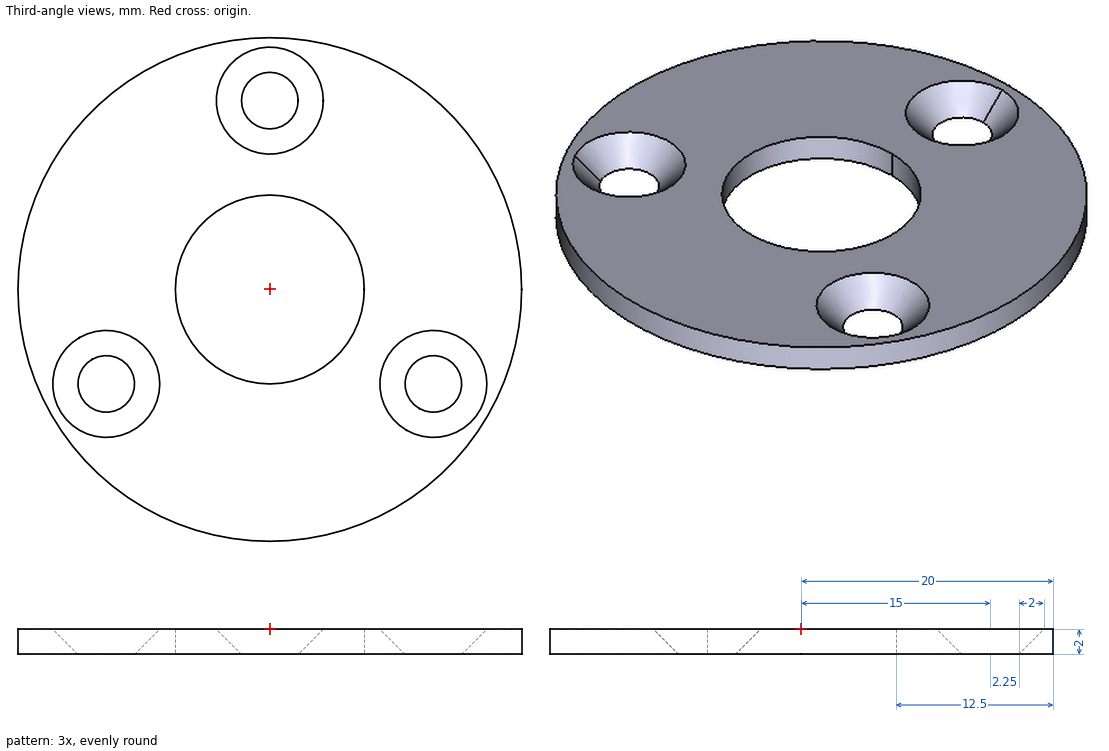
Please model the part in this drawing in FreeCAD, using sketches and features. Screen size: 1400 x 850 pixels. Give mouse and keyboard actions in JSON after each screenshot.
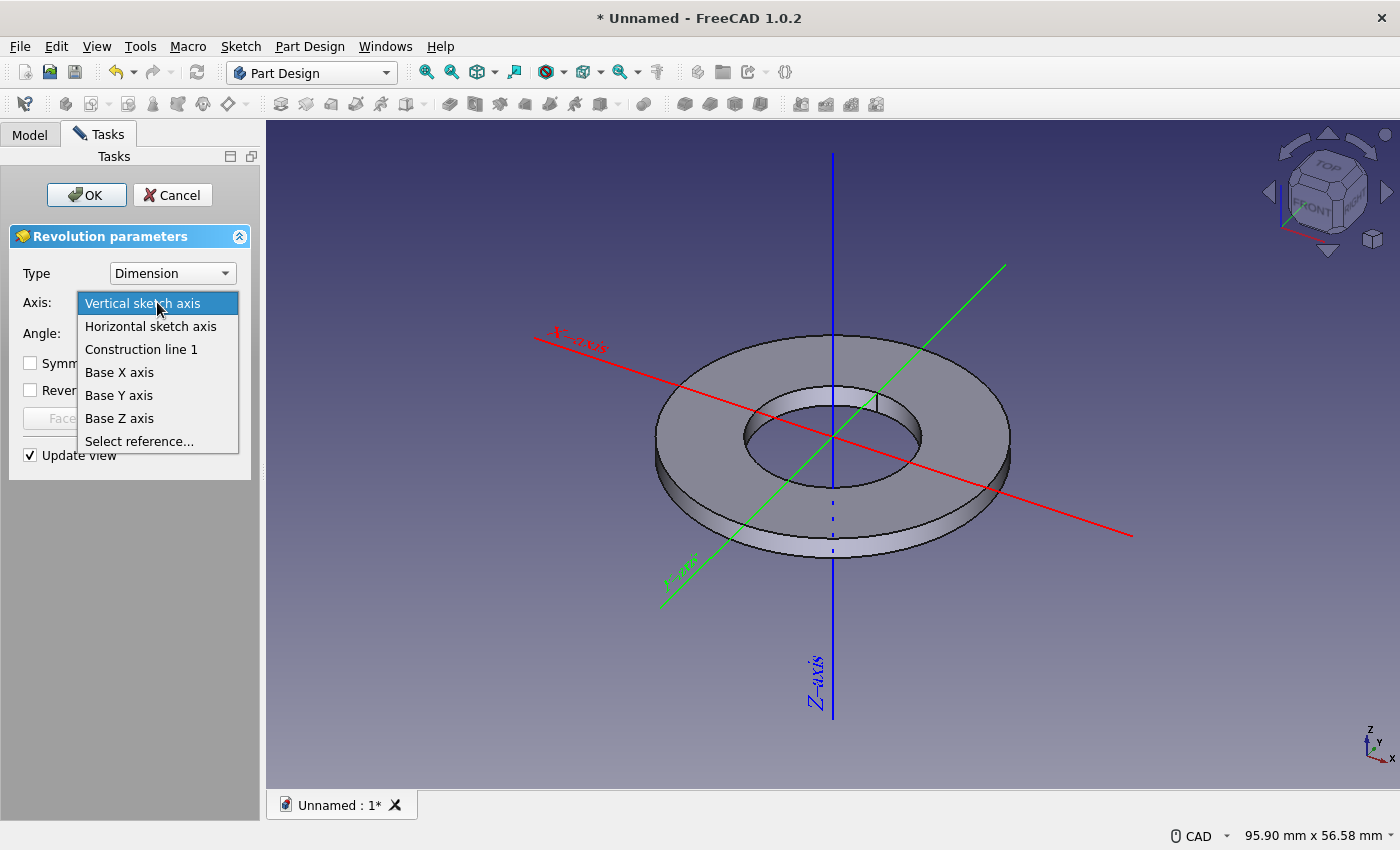
{"action": "left_click", "coordinate": [156, 350]}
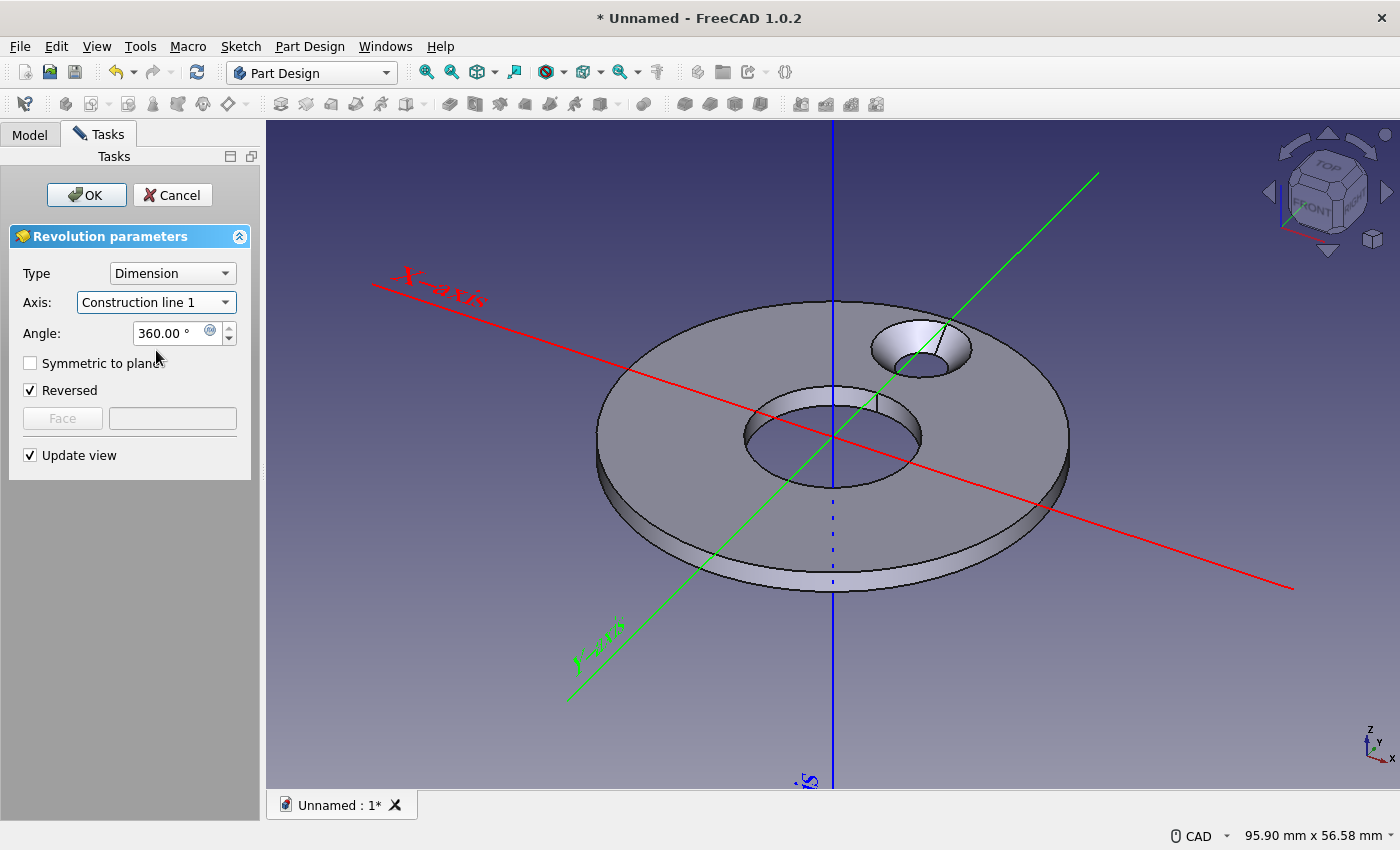
{"action": "left_click", "coordinate": [87, 195]}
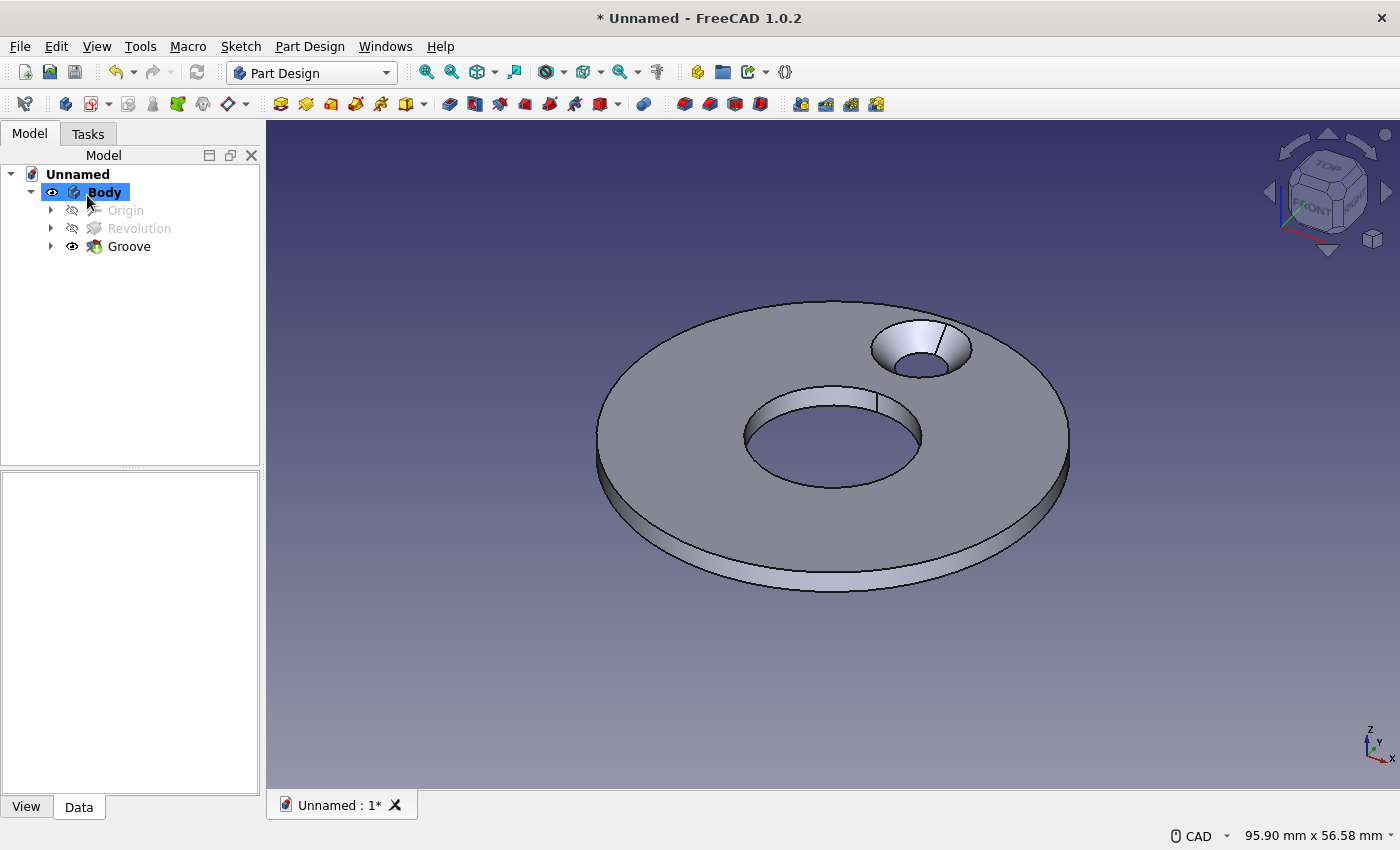
{"action": "left_click", "coordinate": [117, 246]}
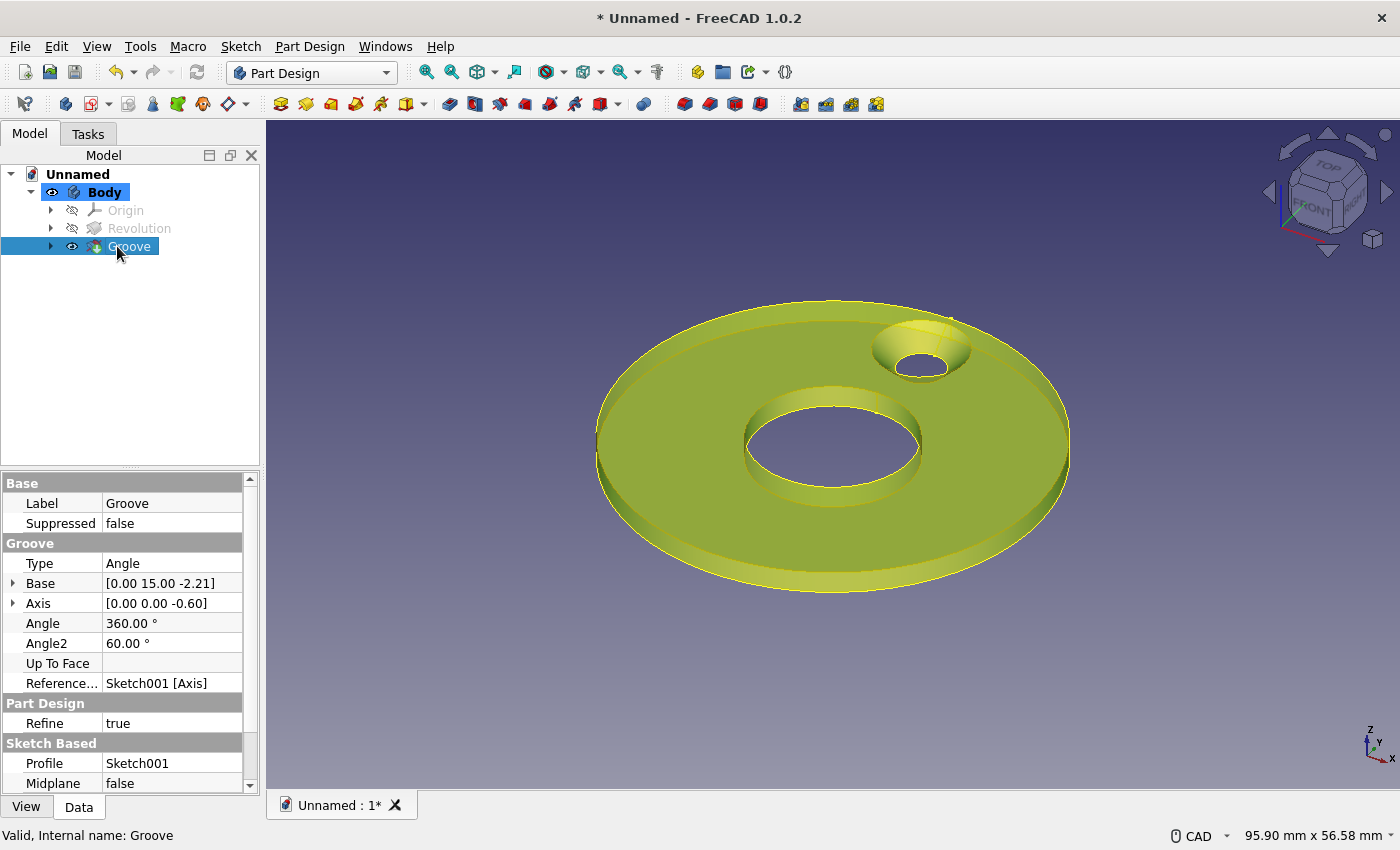
{"action": "left_click", "coordinate": [851, 104]}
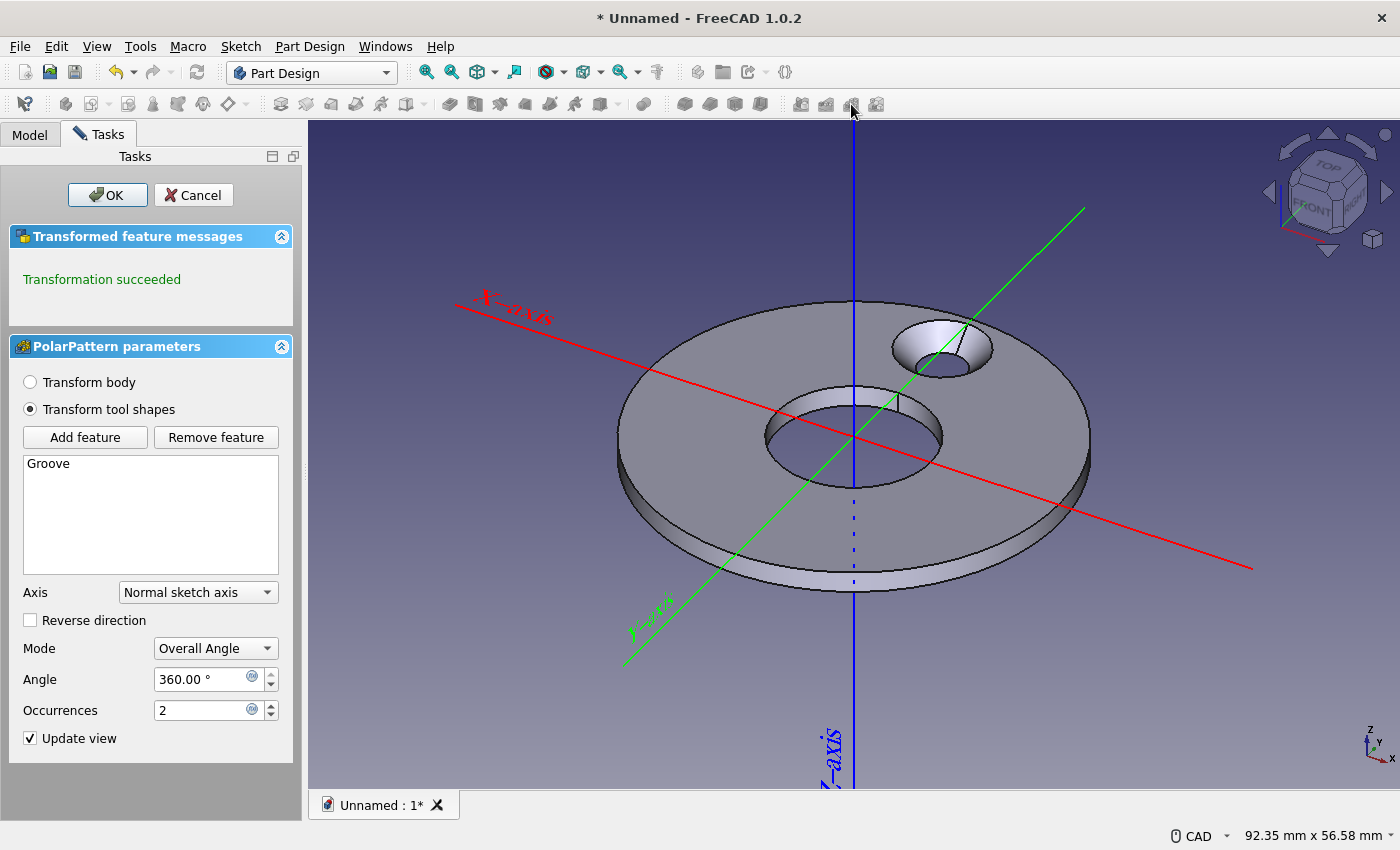
{"action": "left_click", "coordinate": [199, 592]}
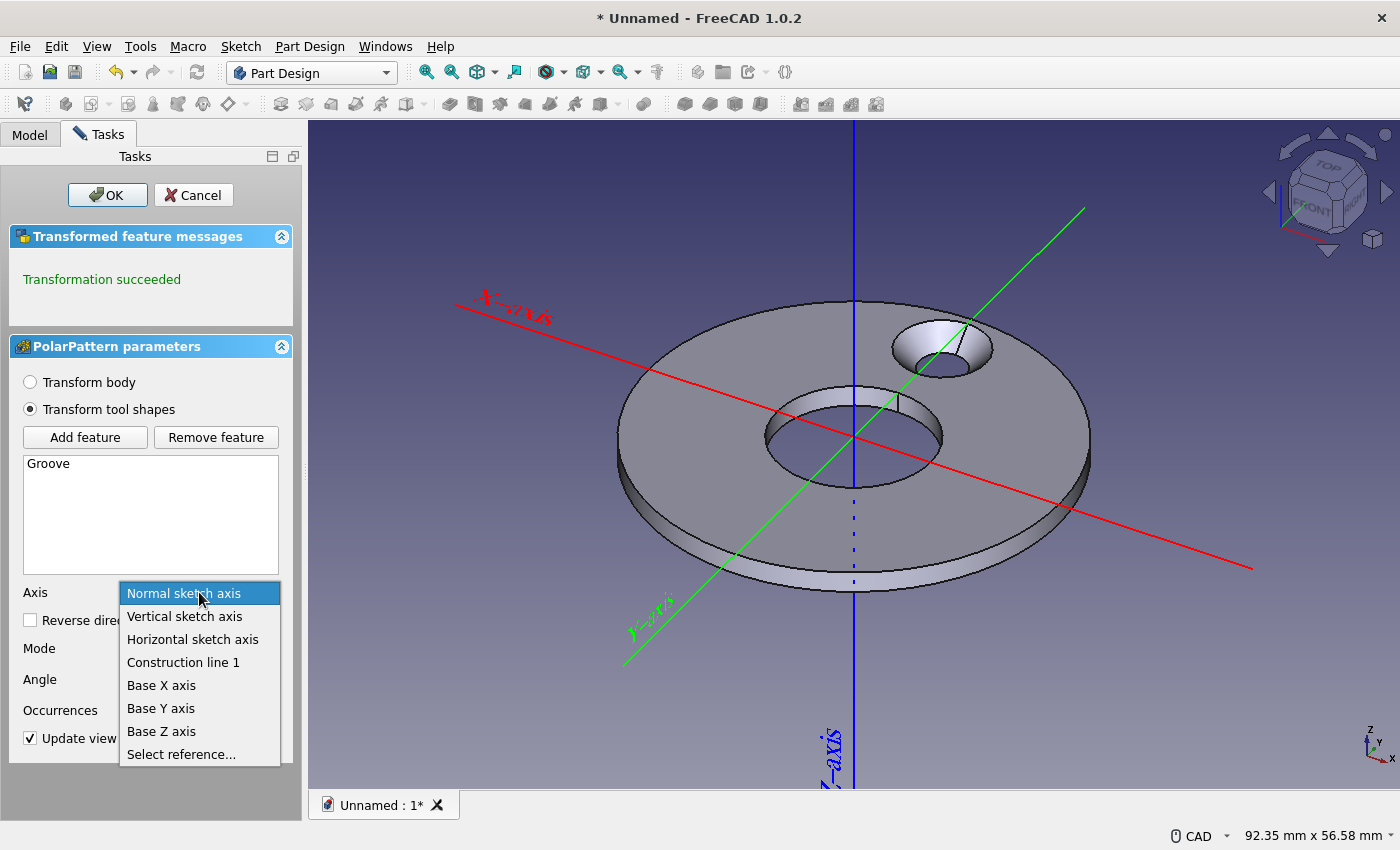
{"action": "left_click", "coordinate": [198, 732]}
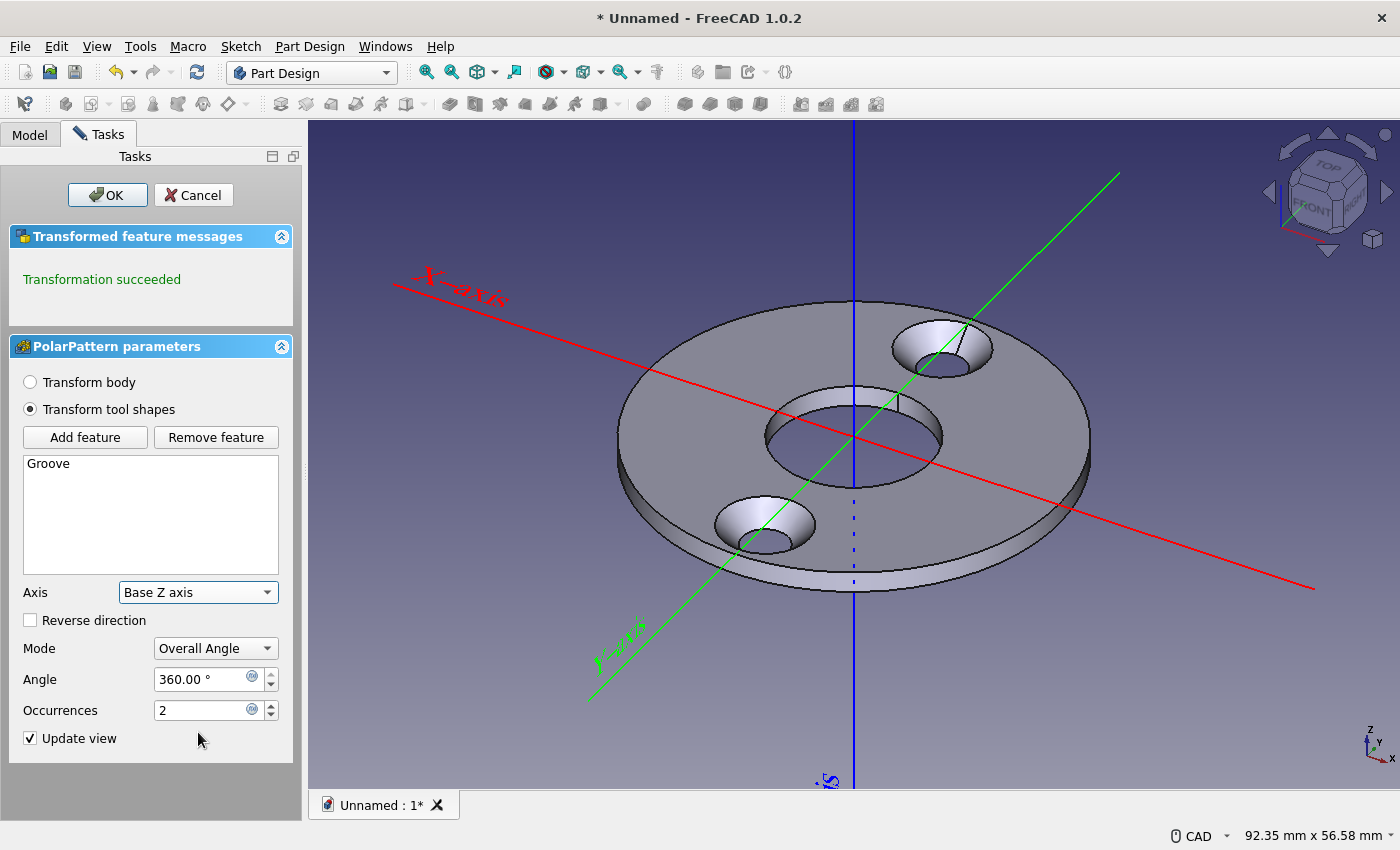
{"action": "triple_click", "coordinate": [210, 710]}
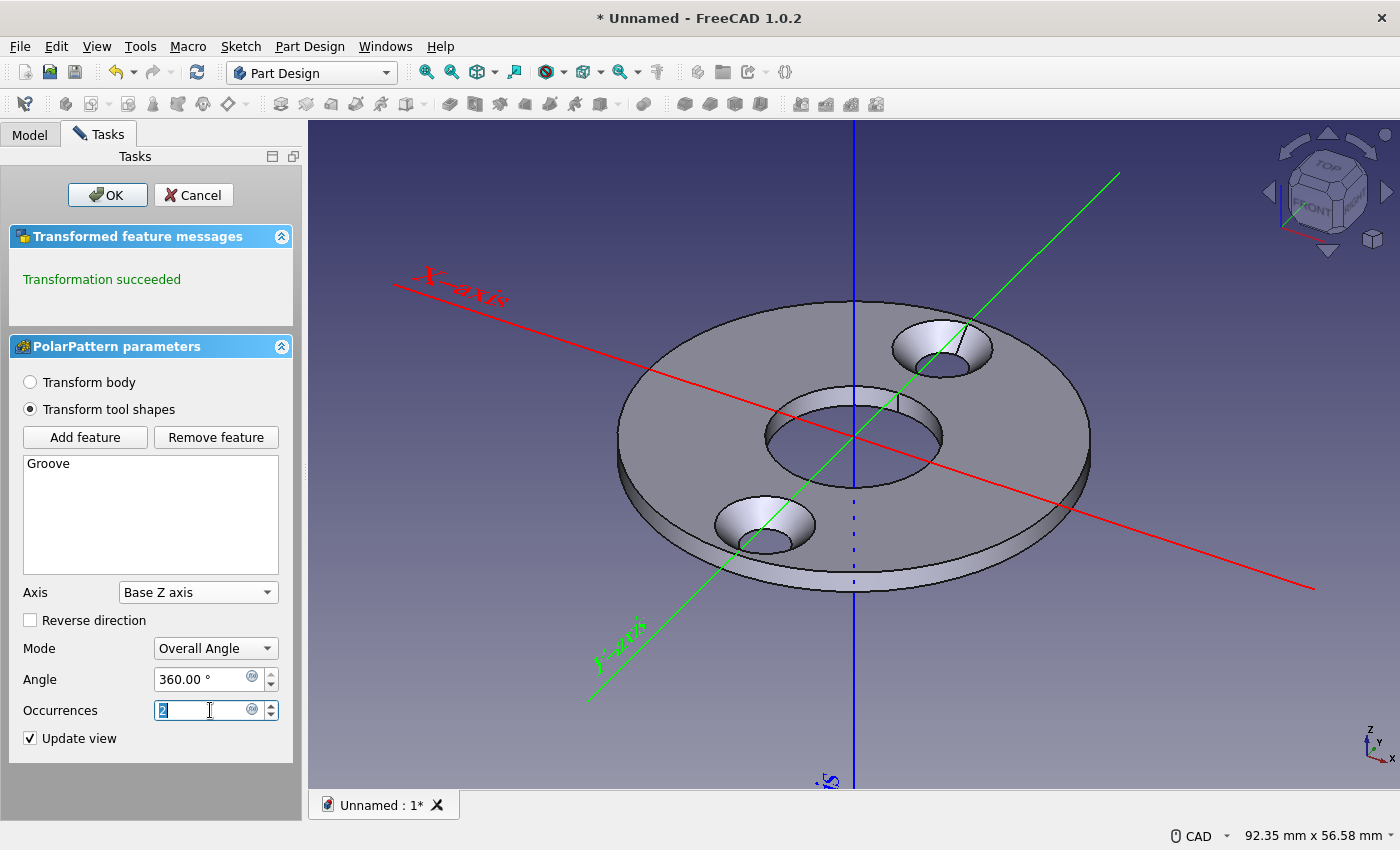
{"action": "type", "text": "3"}
{"action": "key", "text": "Tab"}